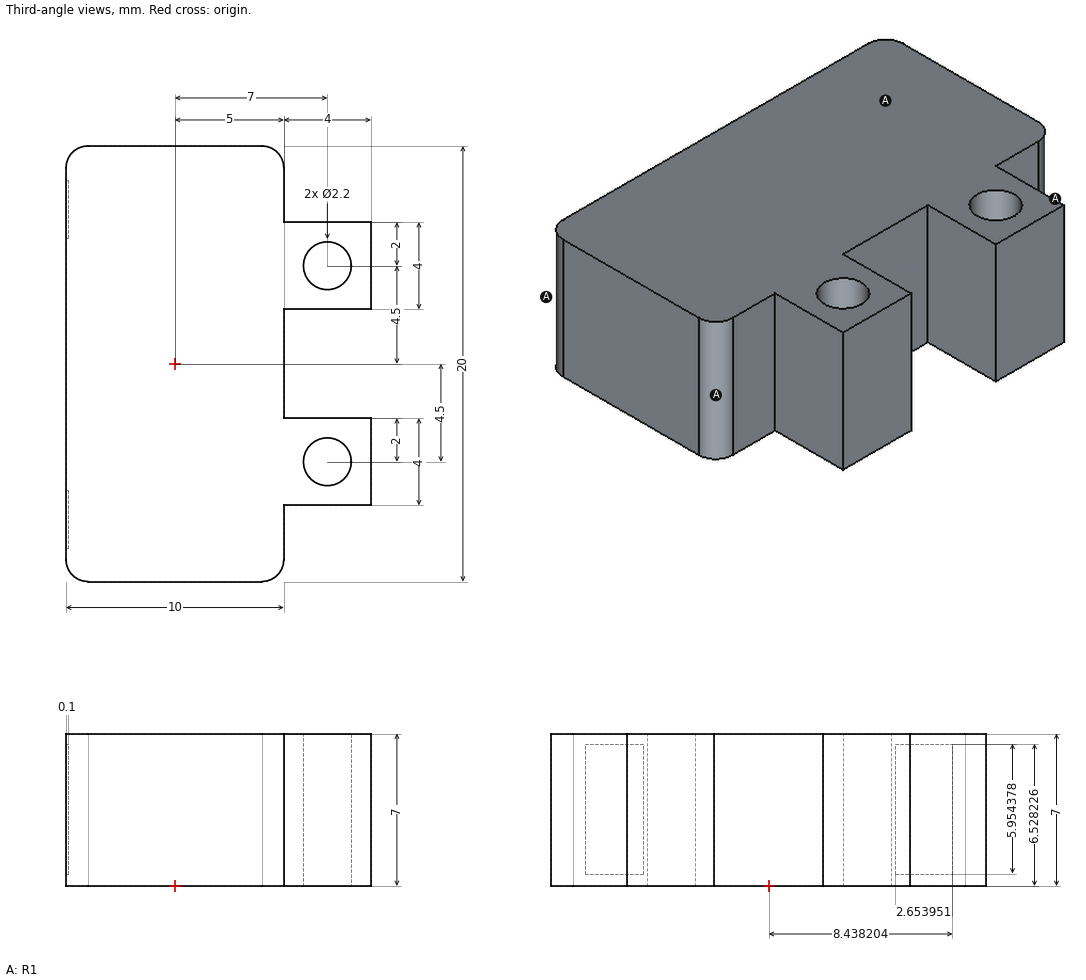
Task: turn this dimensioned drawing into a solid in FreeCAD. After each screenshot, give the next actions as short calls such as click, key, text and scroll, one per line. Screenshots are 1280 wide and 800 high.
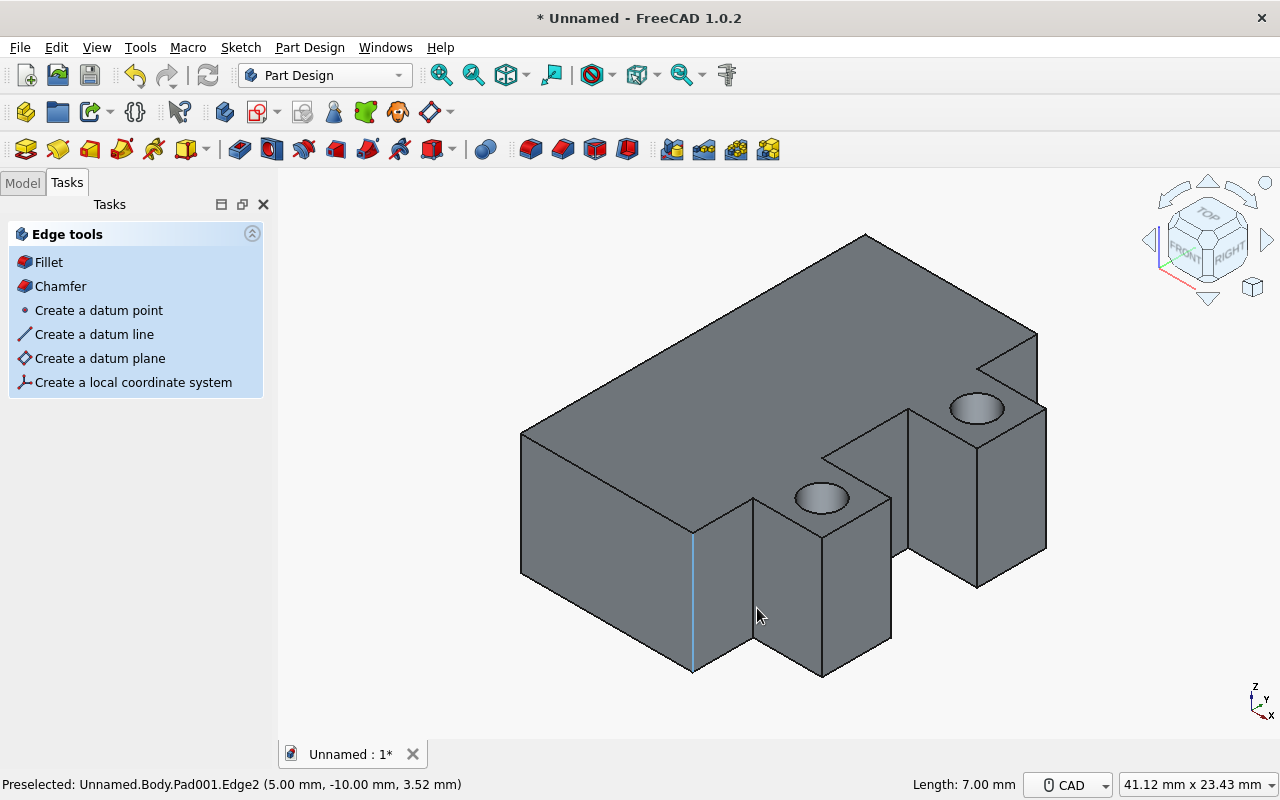
key(2)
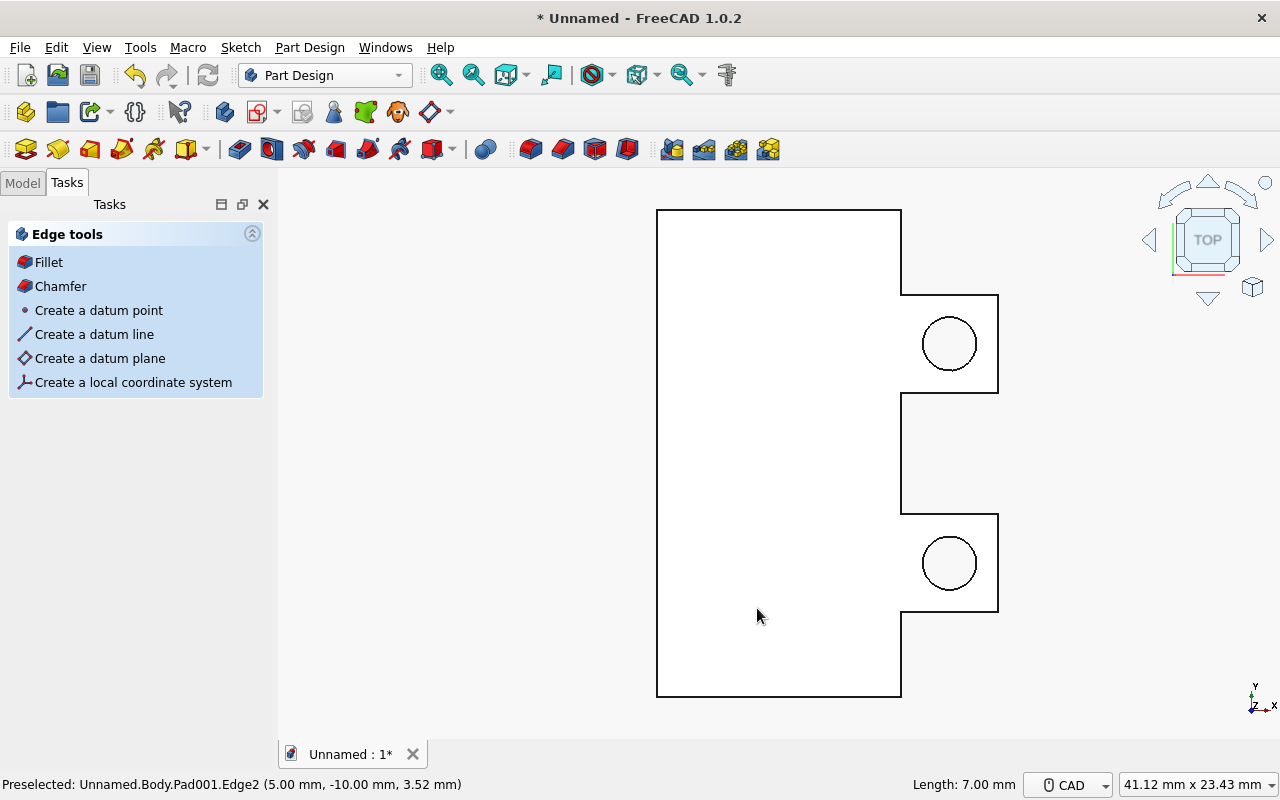
key(1)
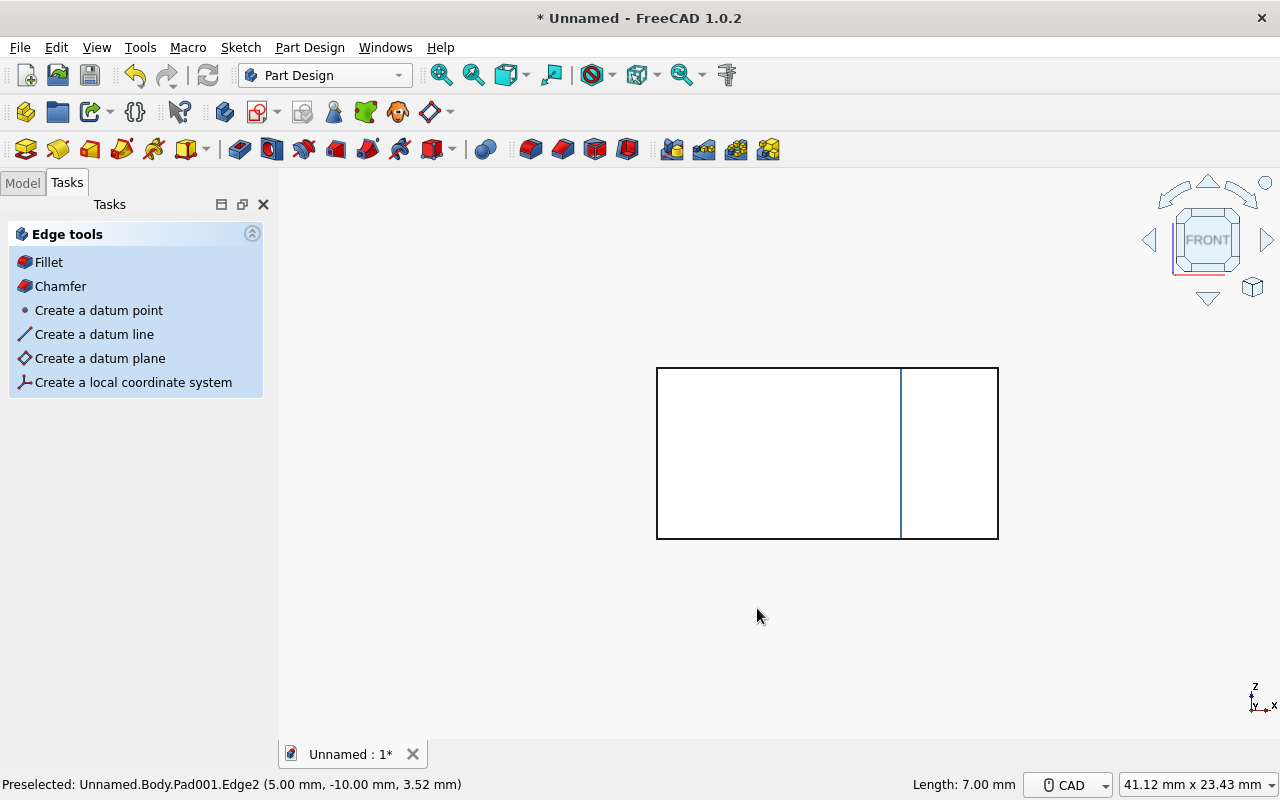
key(v)
key(f)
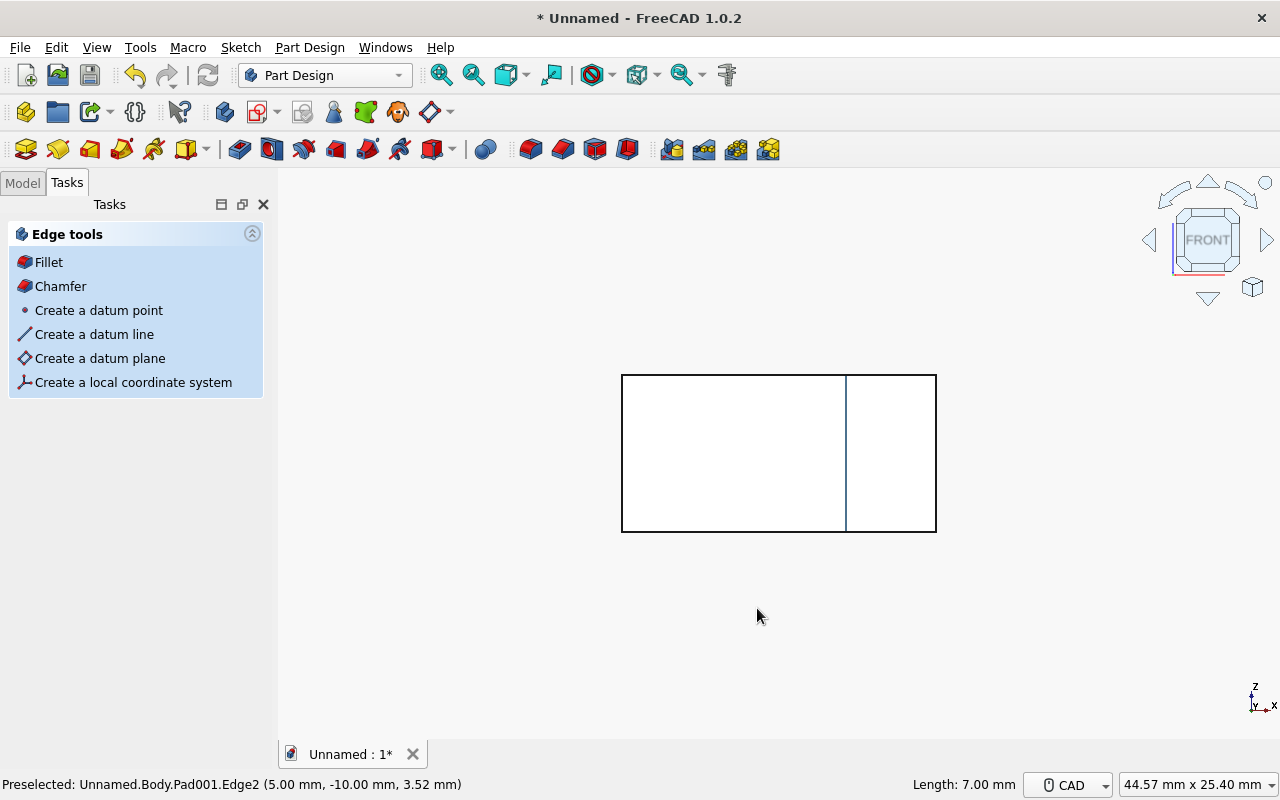
click(622, 453, ctrl)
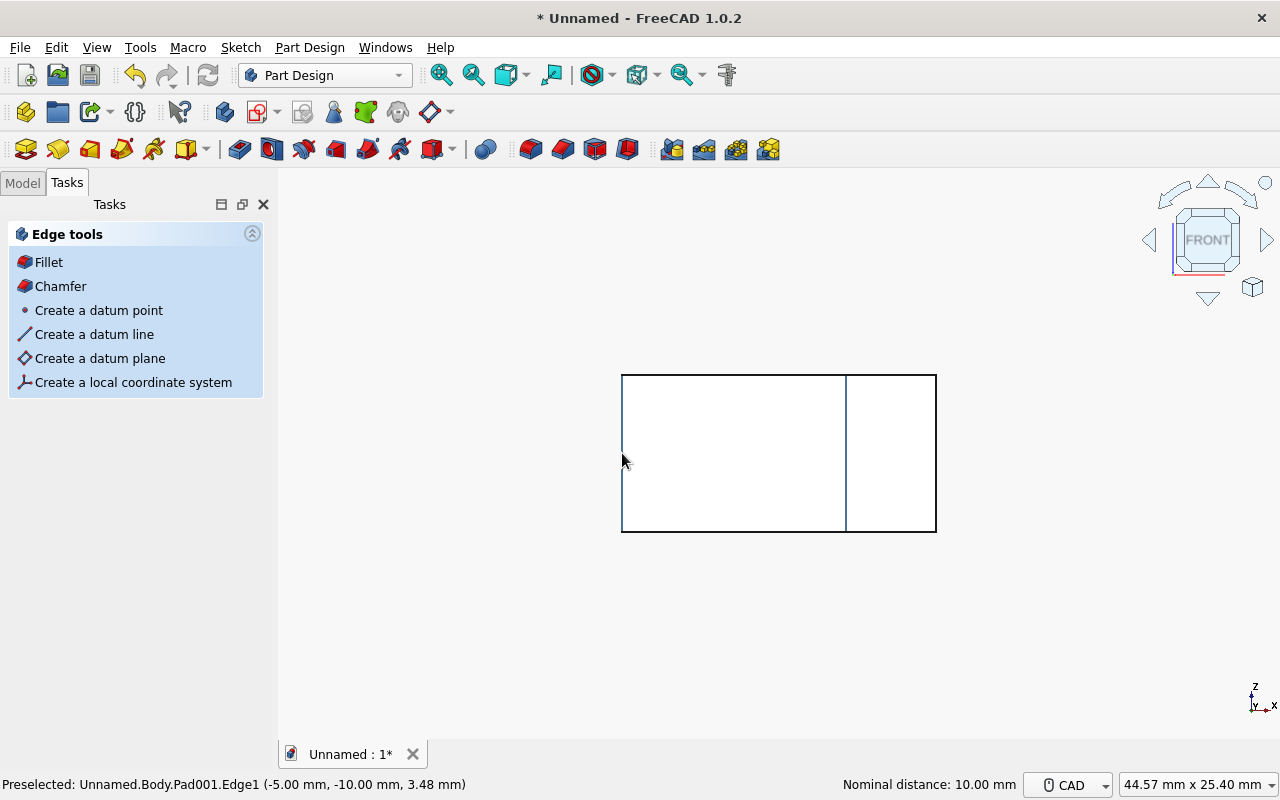
key(3)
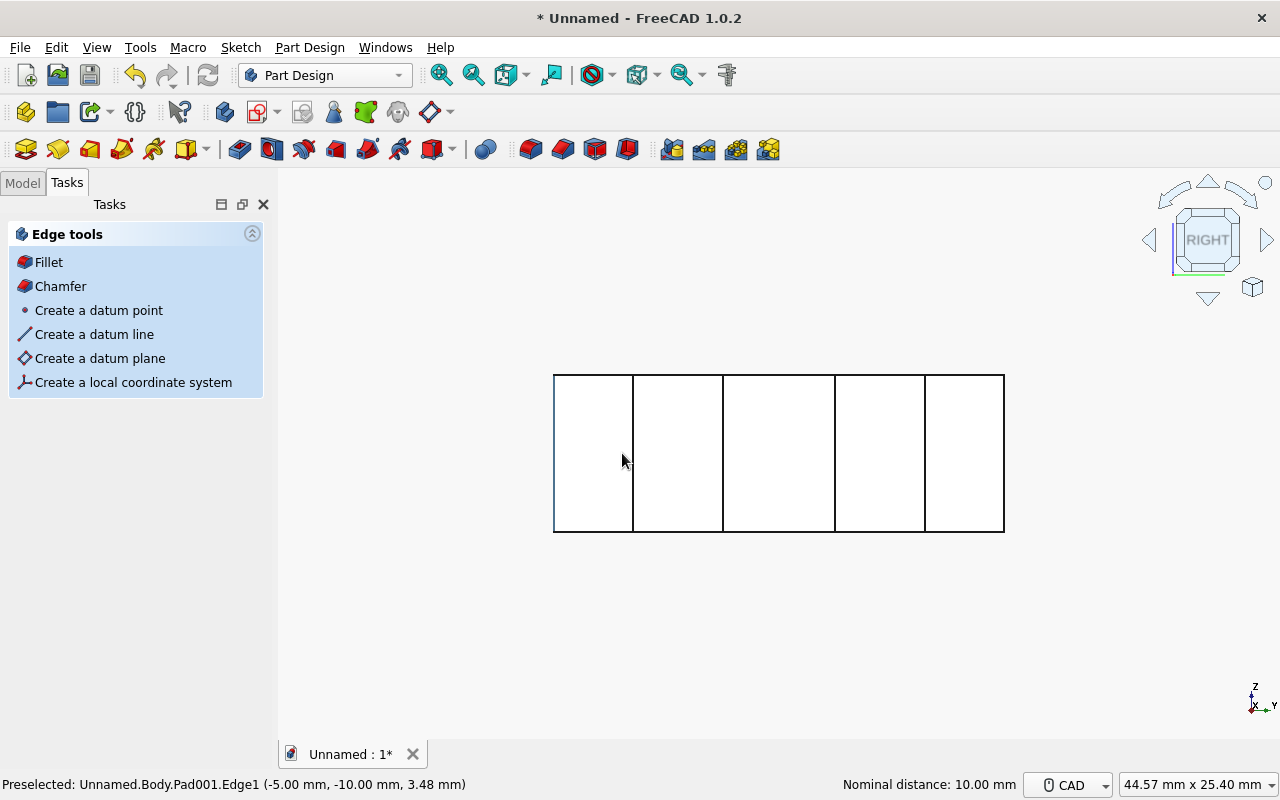
key(v)
key(f)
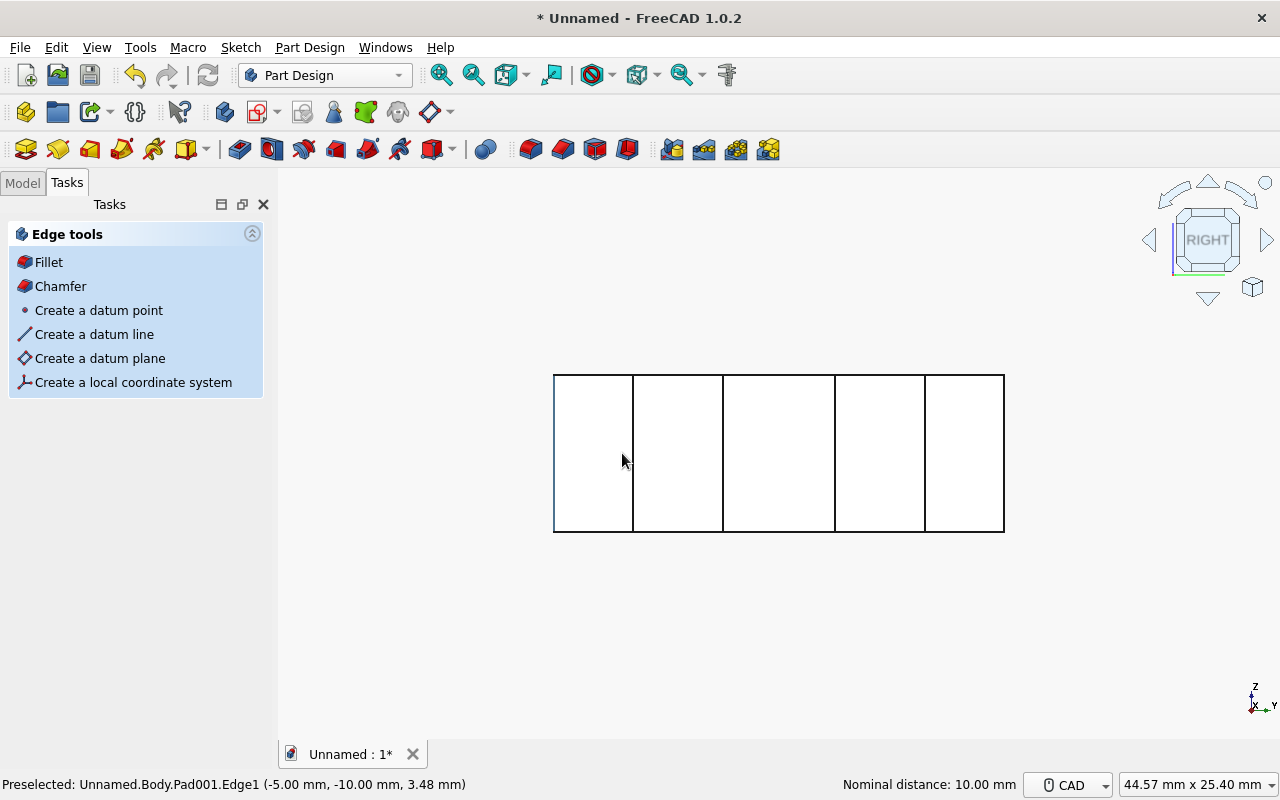
click(1004, 452, ctrl)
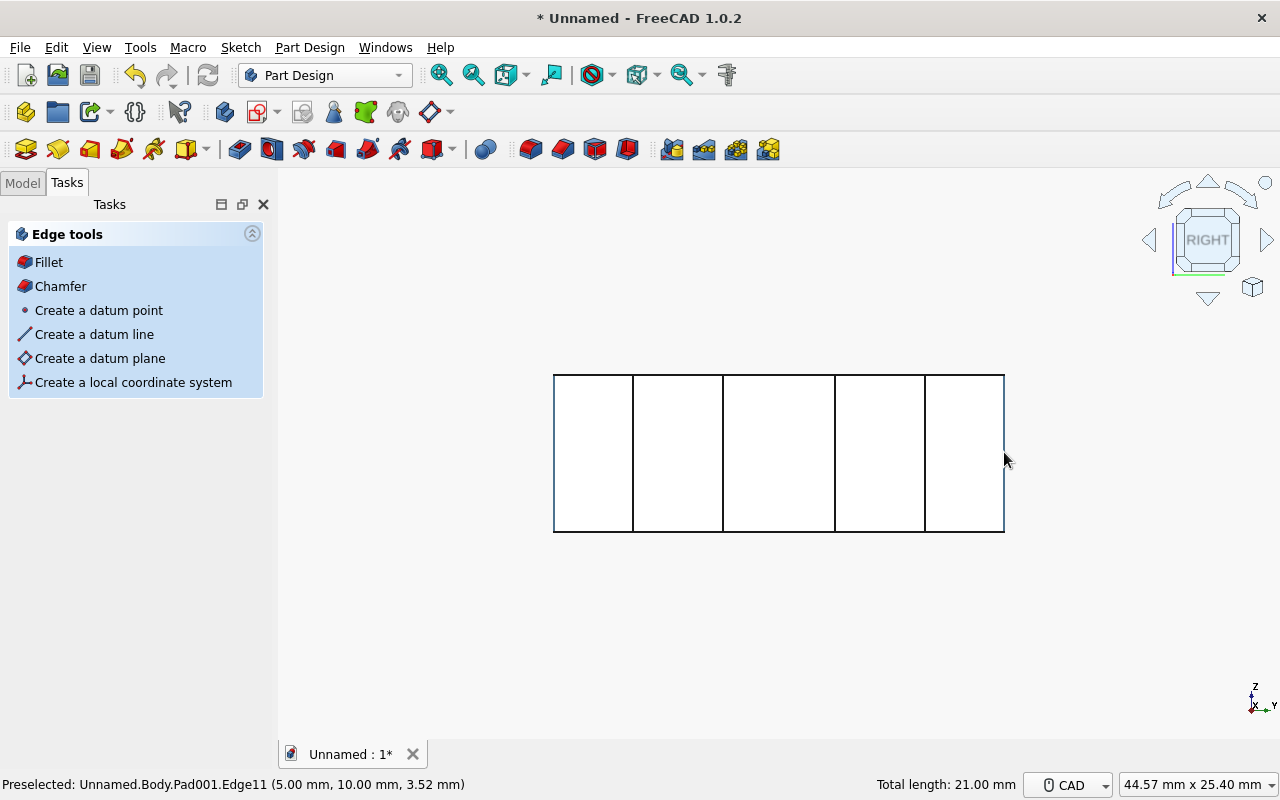
key(5)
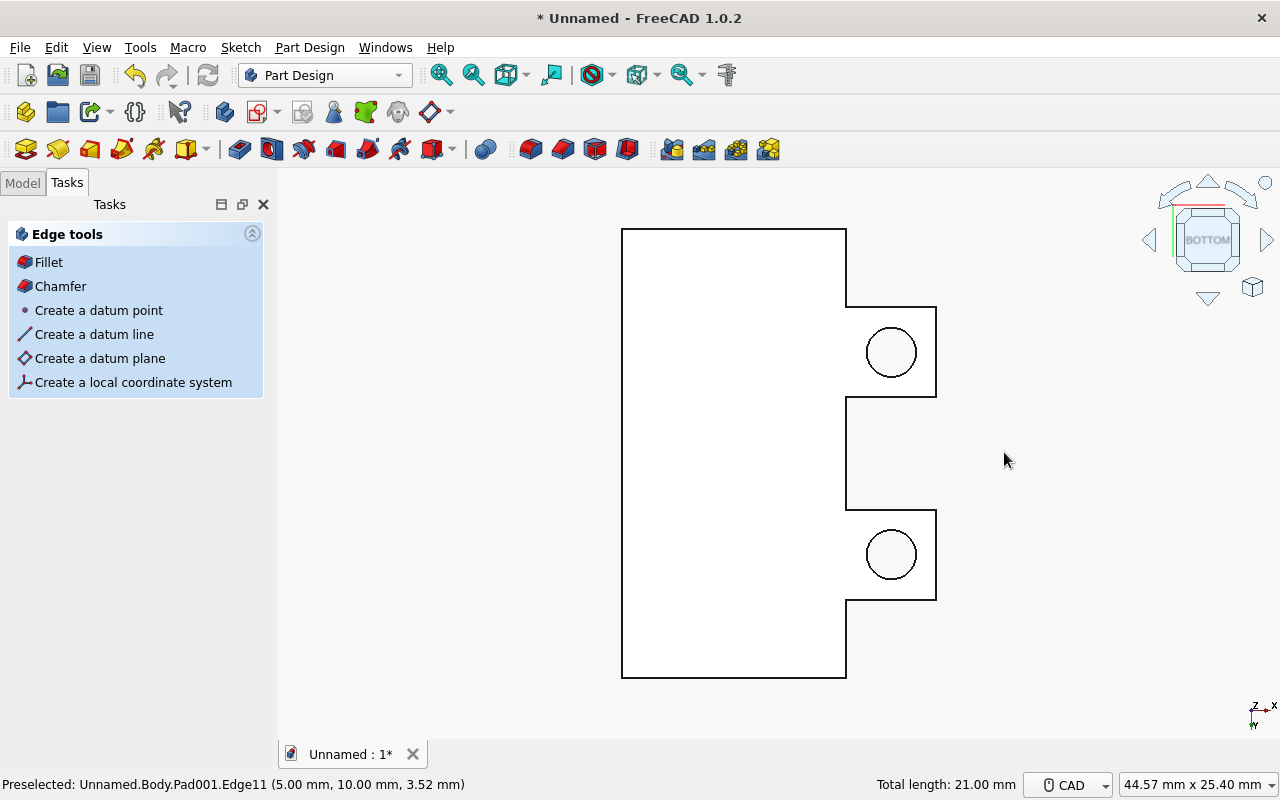
key(4)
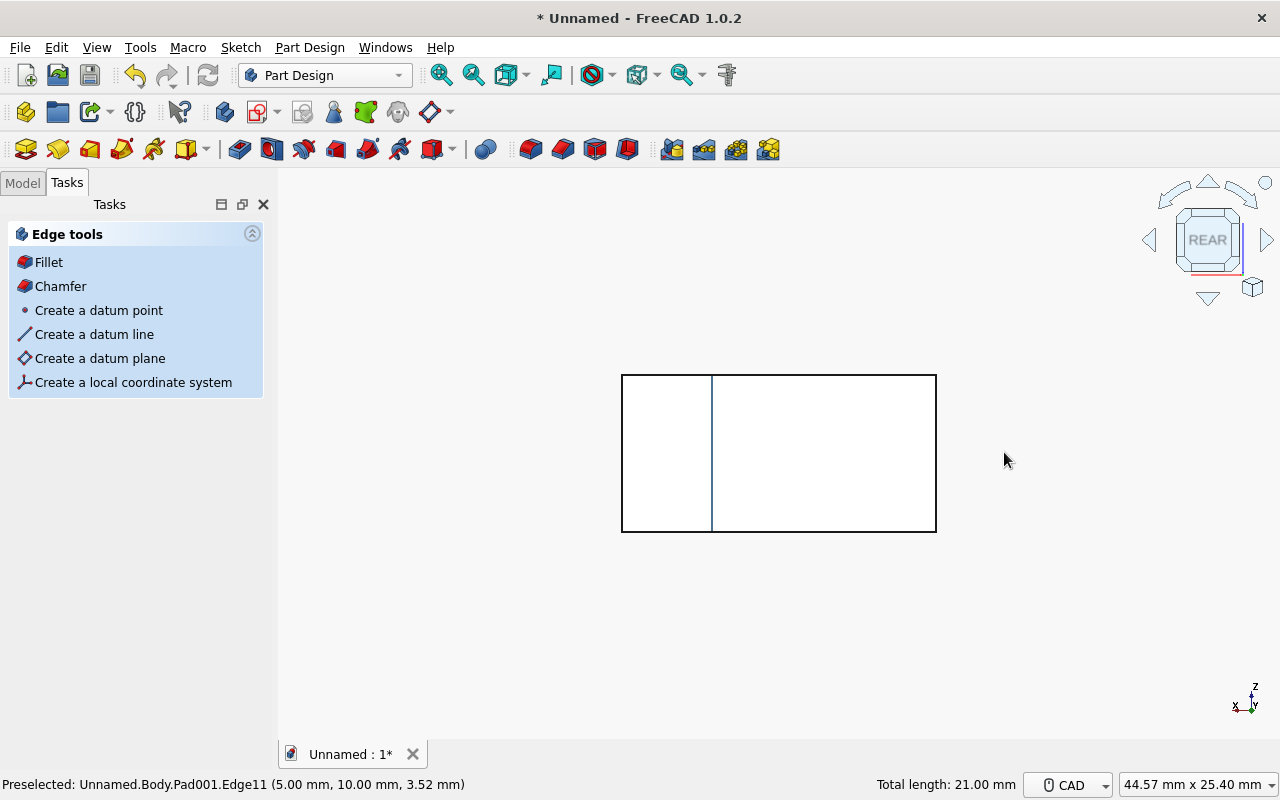
click(442, 76)